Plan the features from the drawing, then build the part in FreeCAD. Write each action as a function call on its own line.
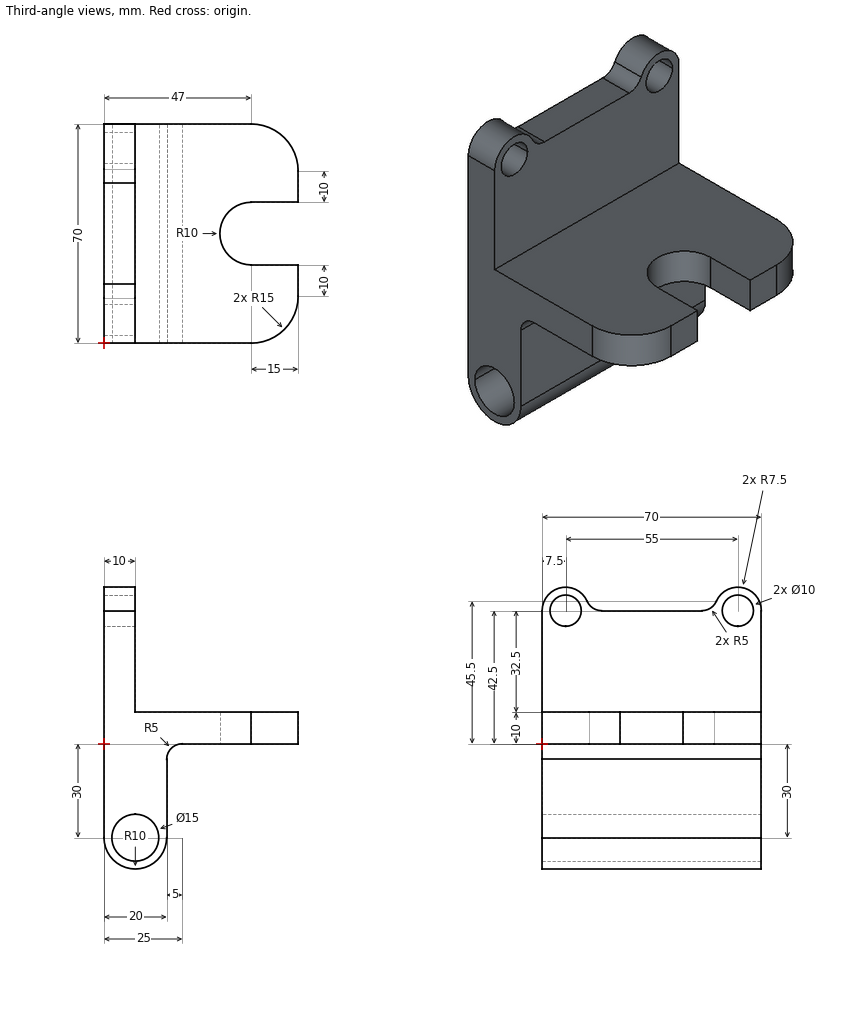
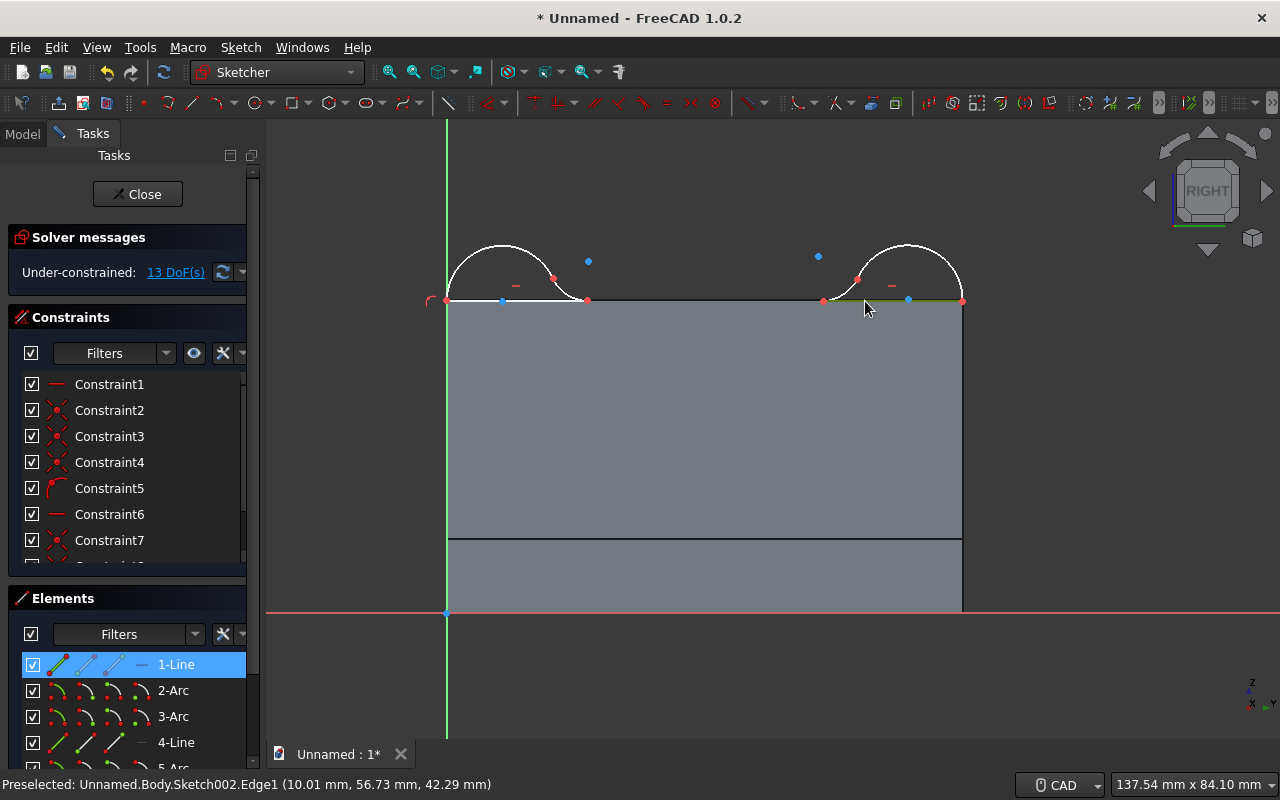
click(850, 289)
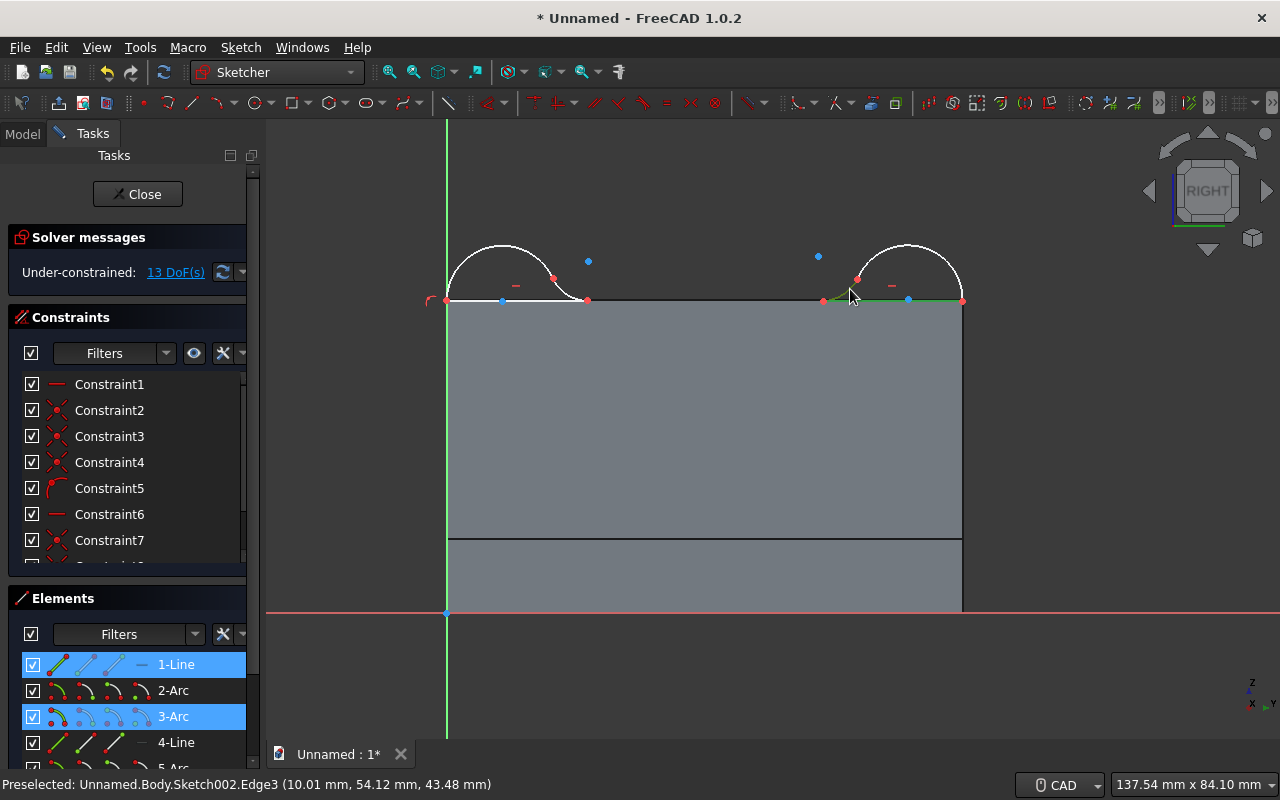
click(644, 104)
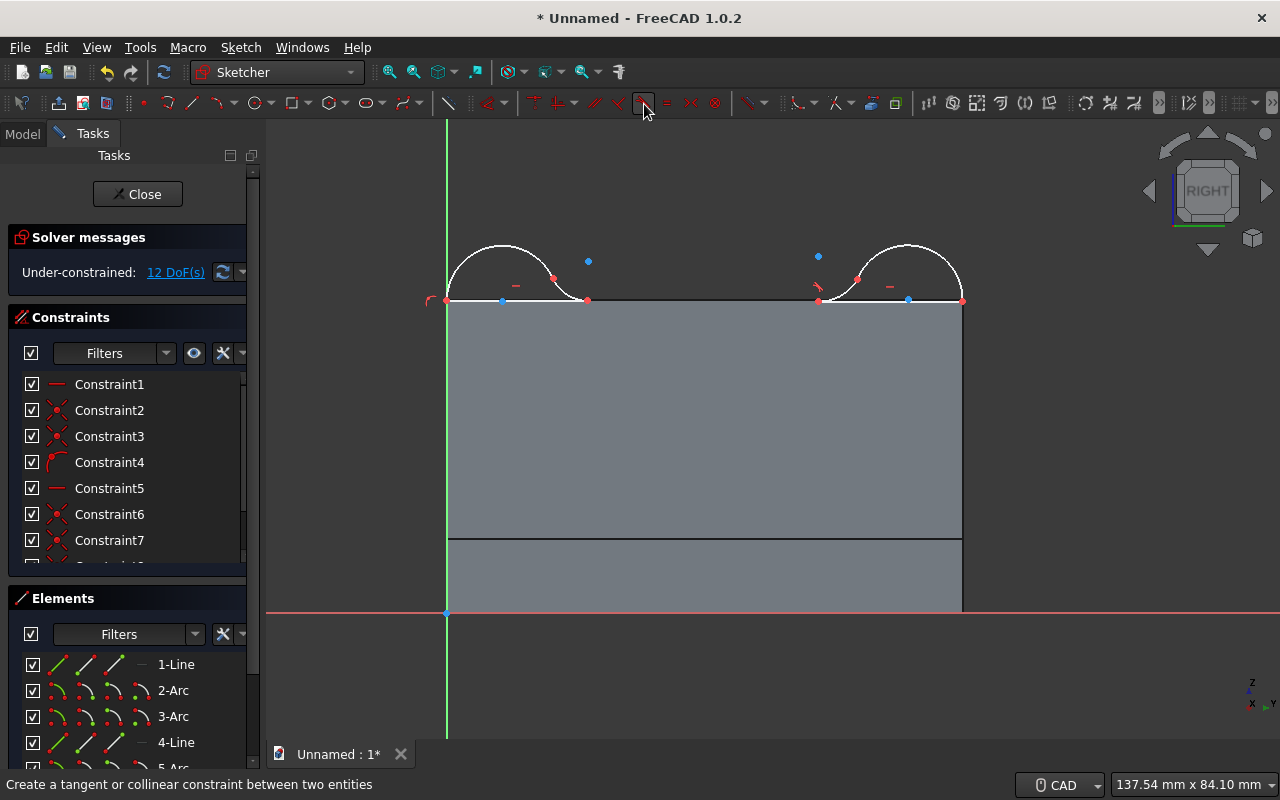
click(946, 261)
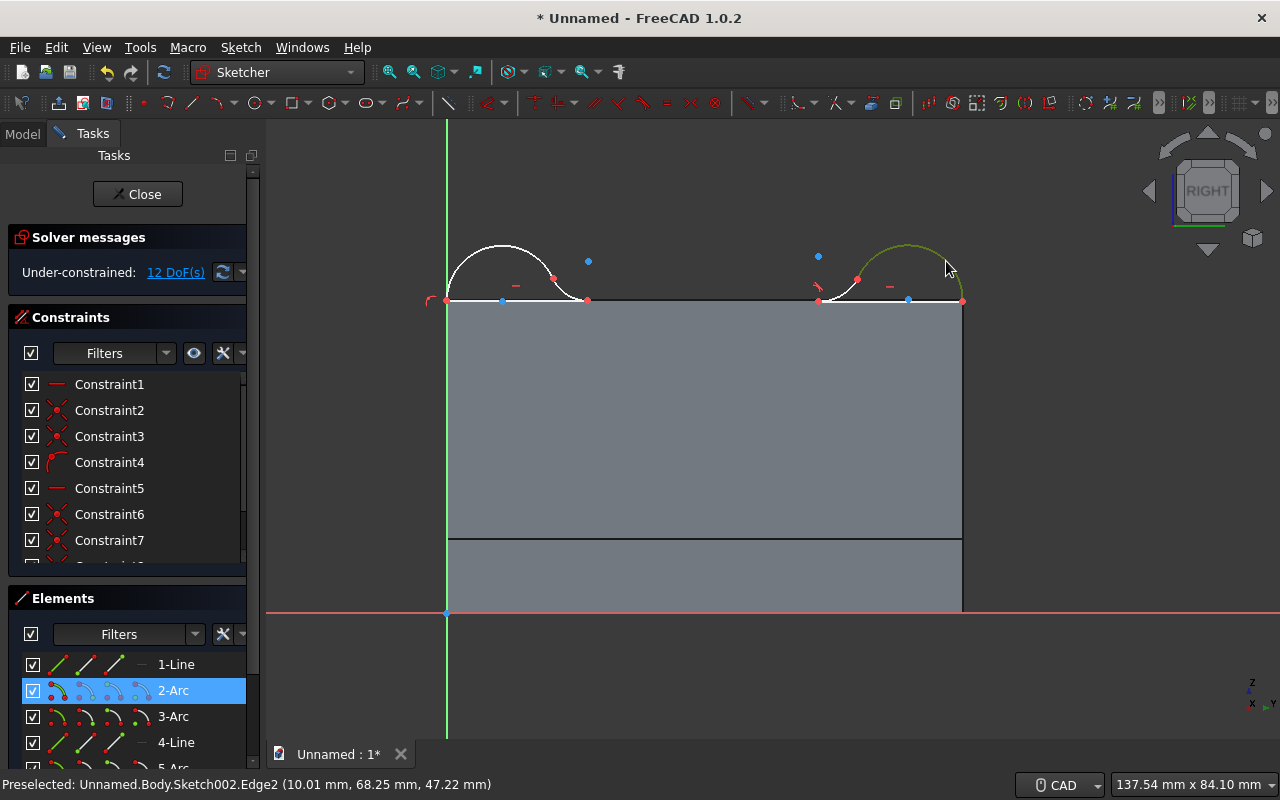
click(849, 290)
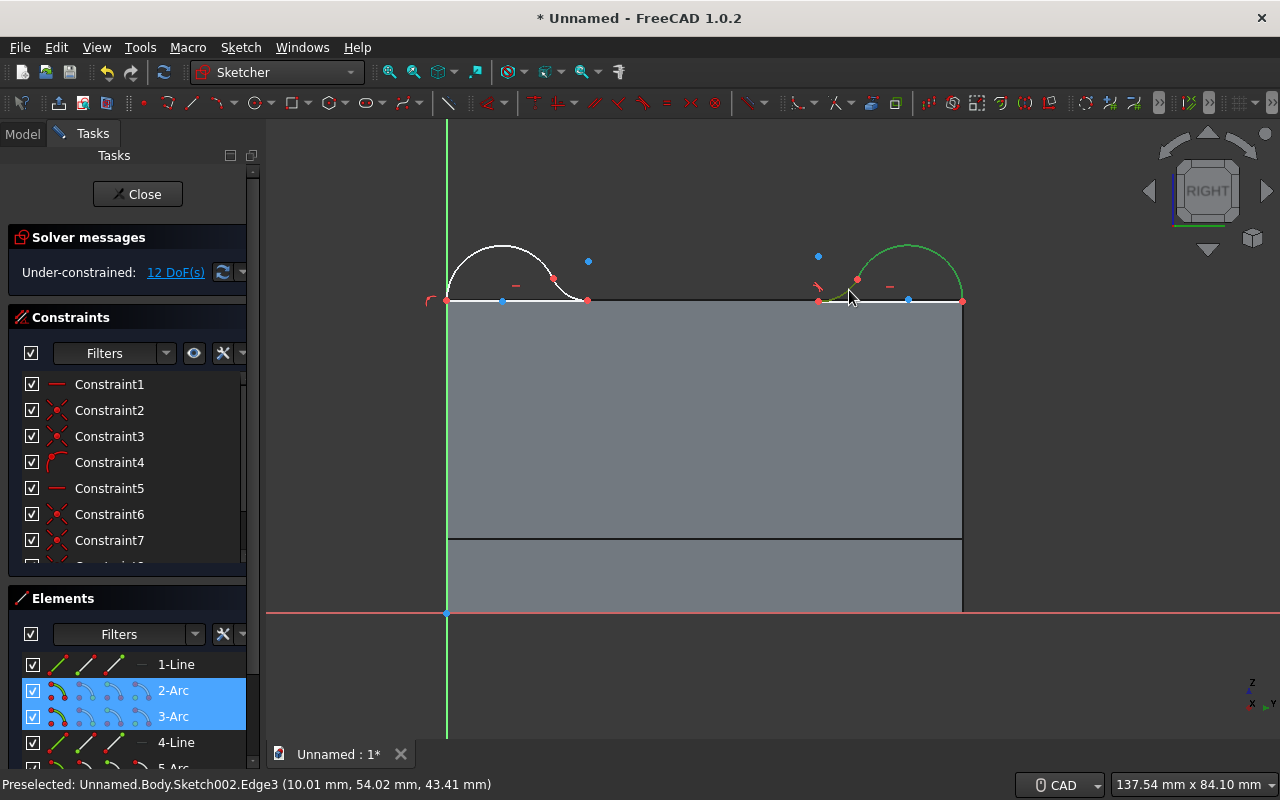
click(644, 104)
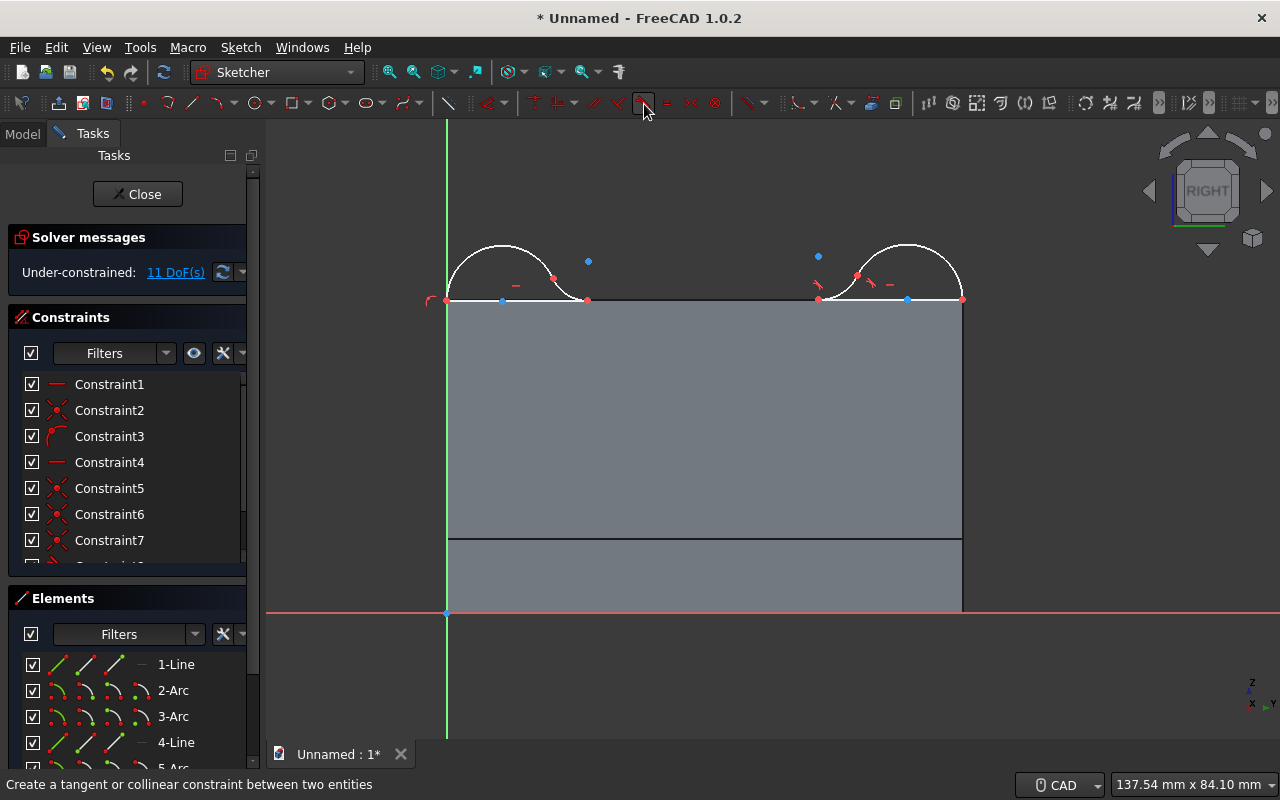
click(489, 301)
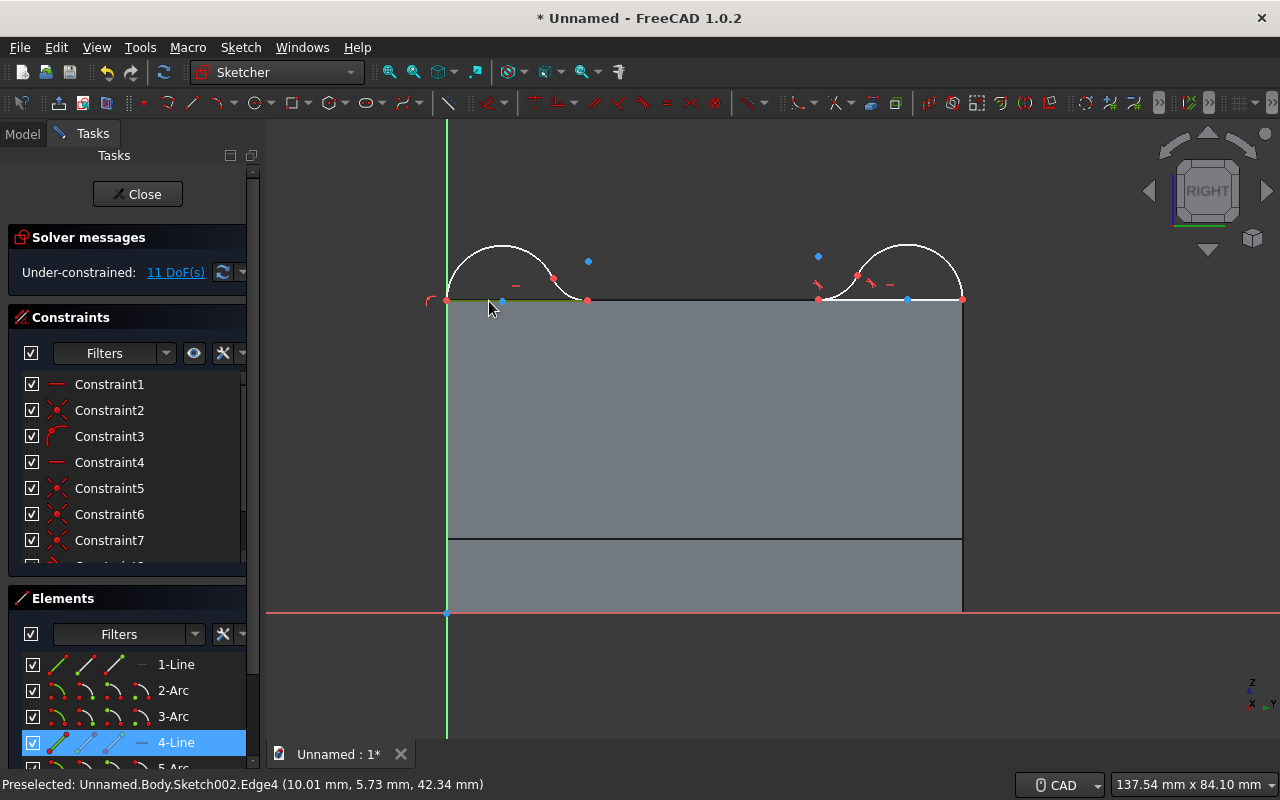
click(560, 289)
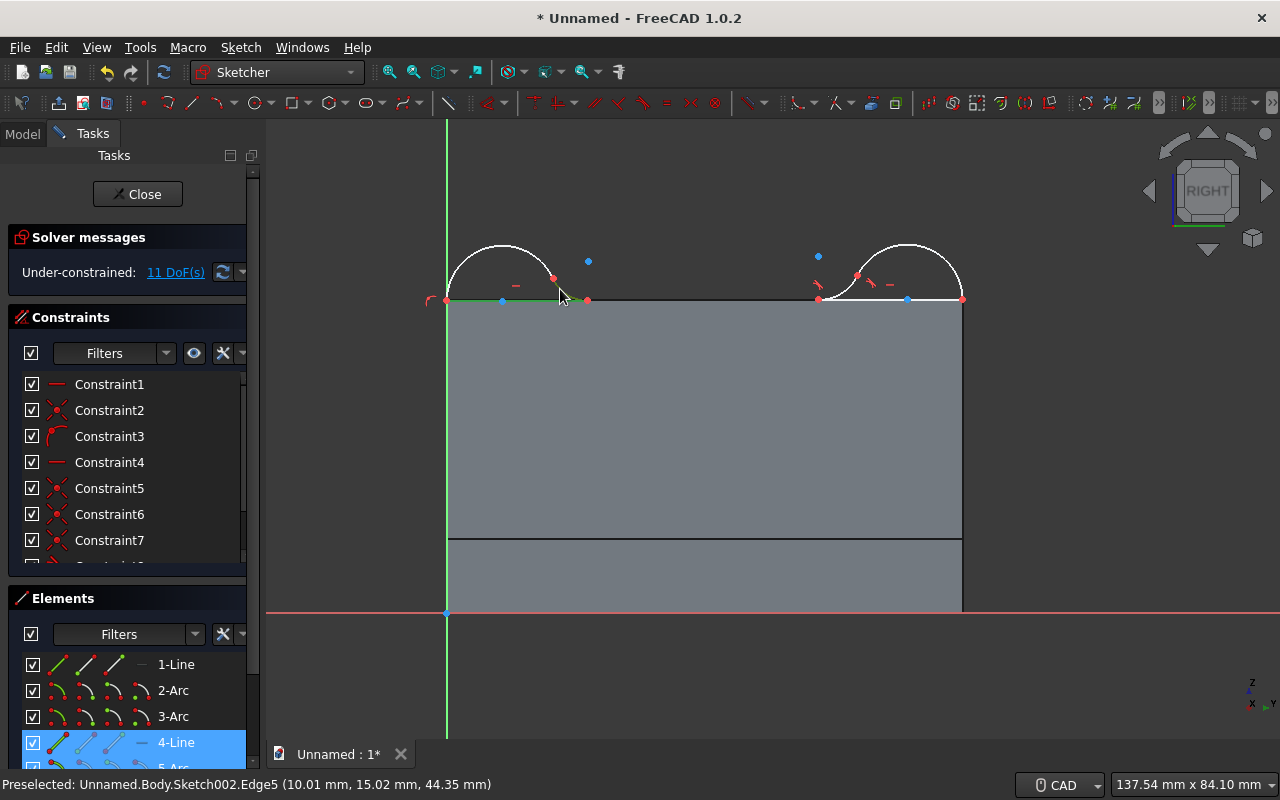
click(644, 104)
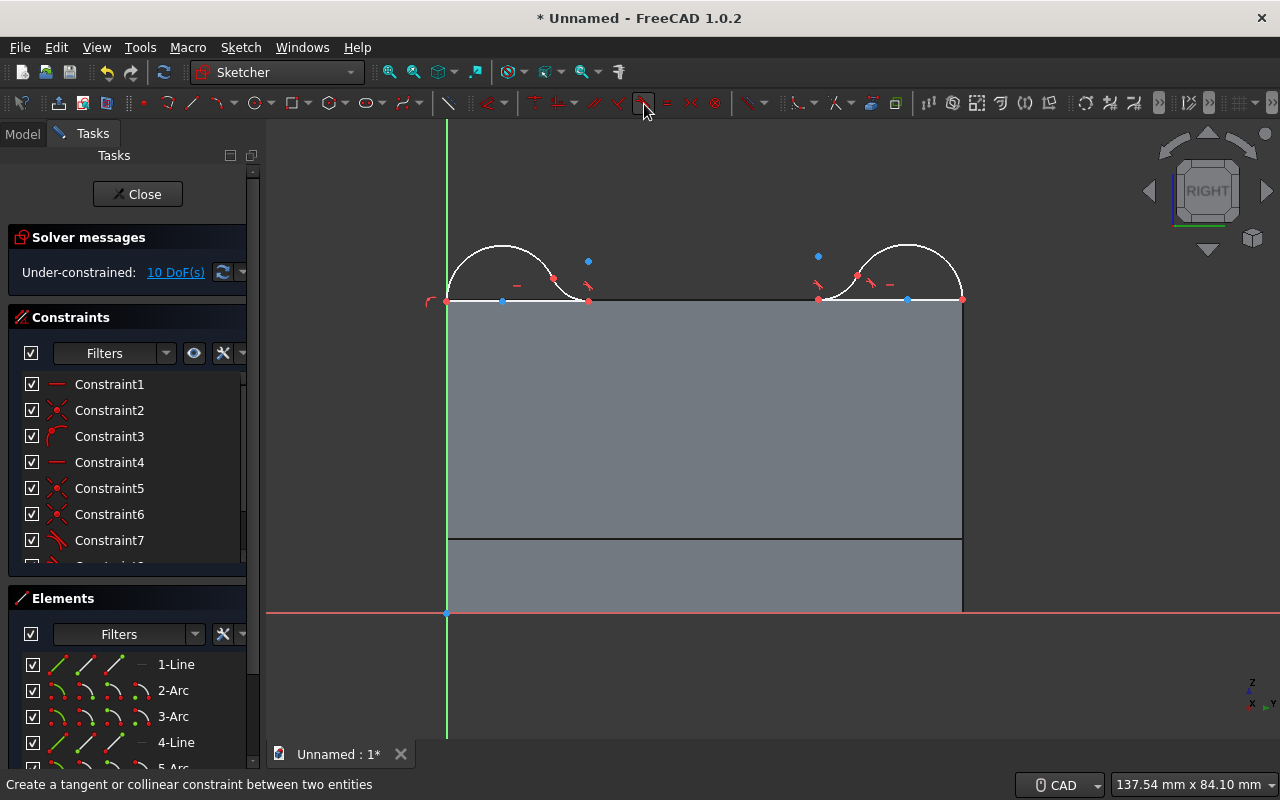
click(561, 290)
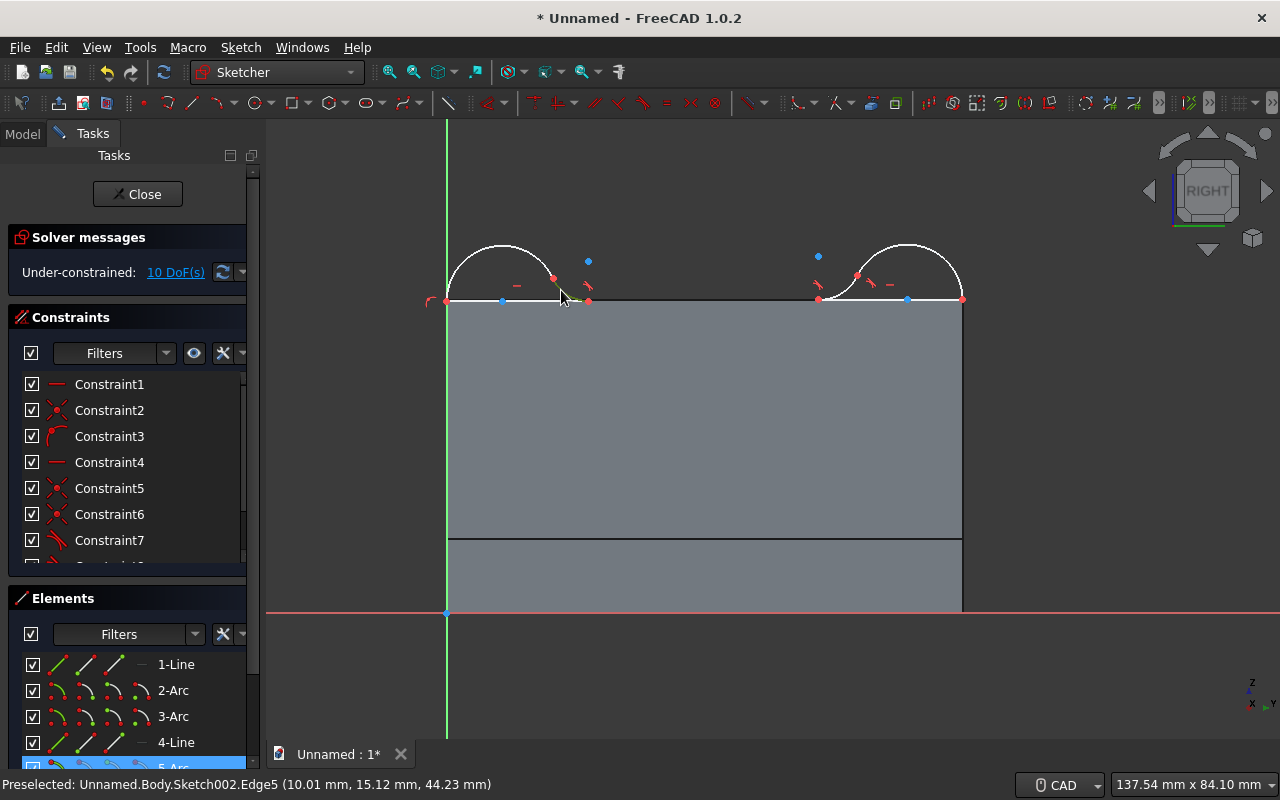
click(521, 249)